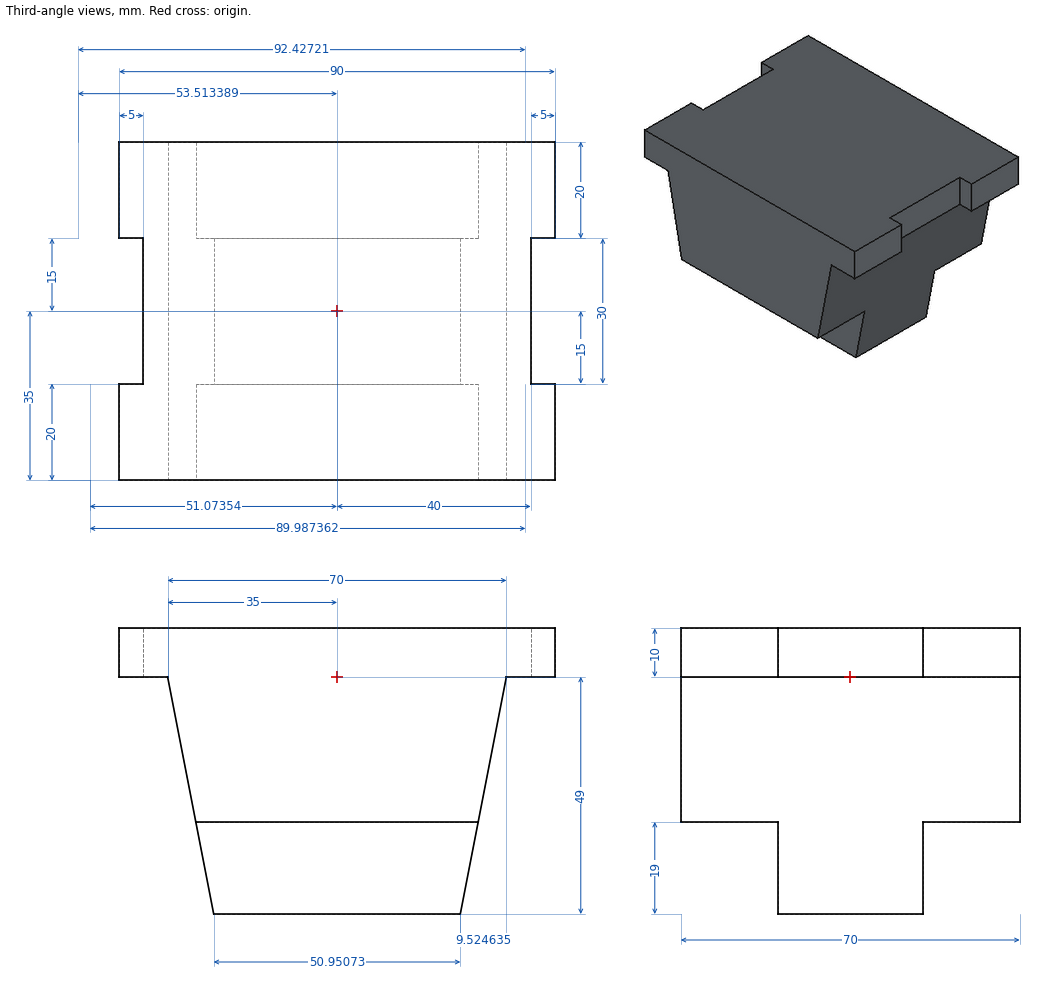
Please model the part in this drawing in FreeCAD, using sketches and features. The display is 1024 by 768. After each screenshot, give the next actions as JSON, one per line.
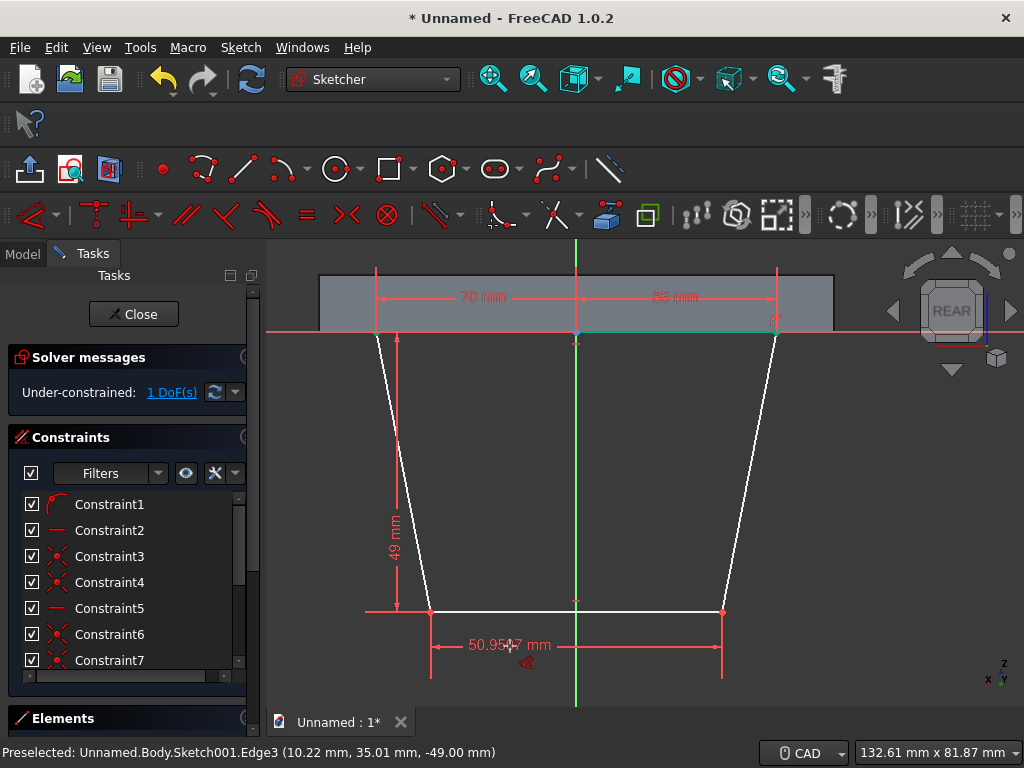
{"action": "left_click", "coordinate": [393, 416]}
{"action": "left_click", "coordinate": [404, 646]}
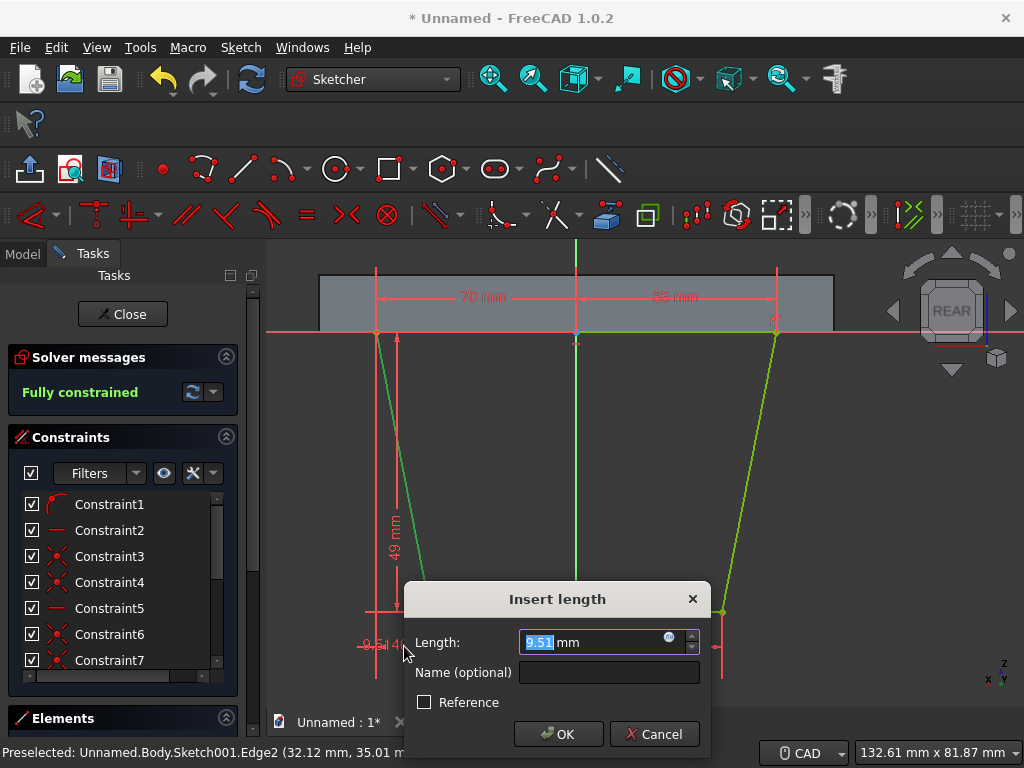
{"action": "type", "text": "9.524635"}
{"action": "key", "text": "Return"}
{"action": "key", "text": "Escape"}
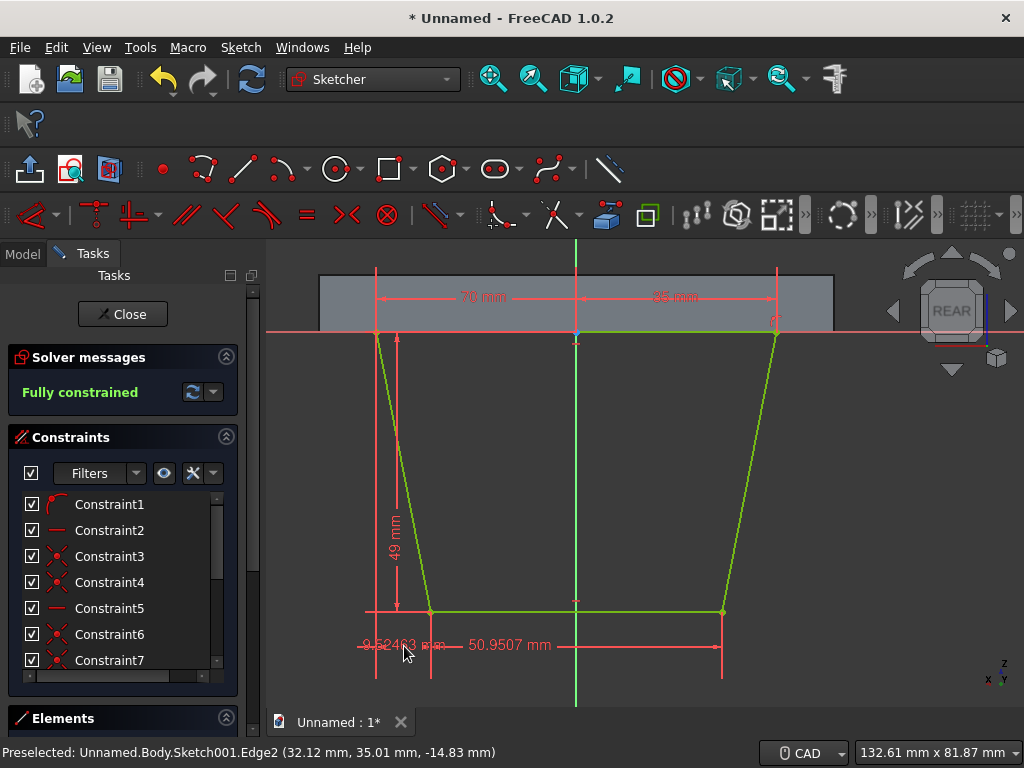
{"action": "left_click", "coordinate": [123, 314]}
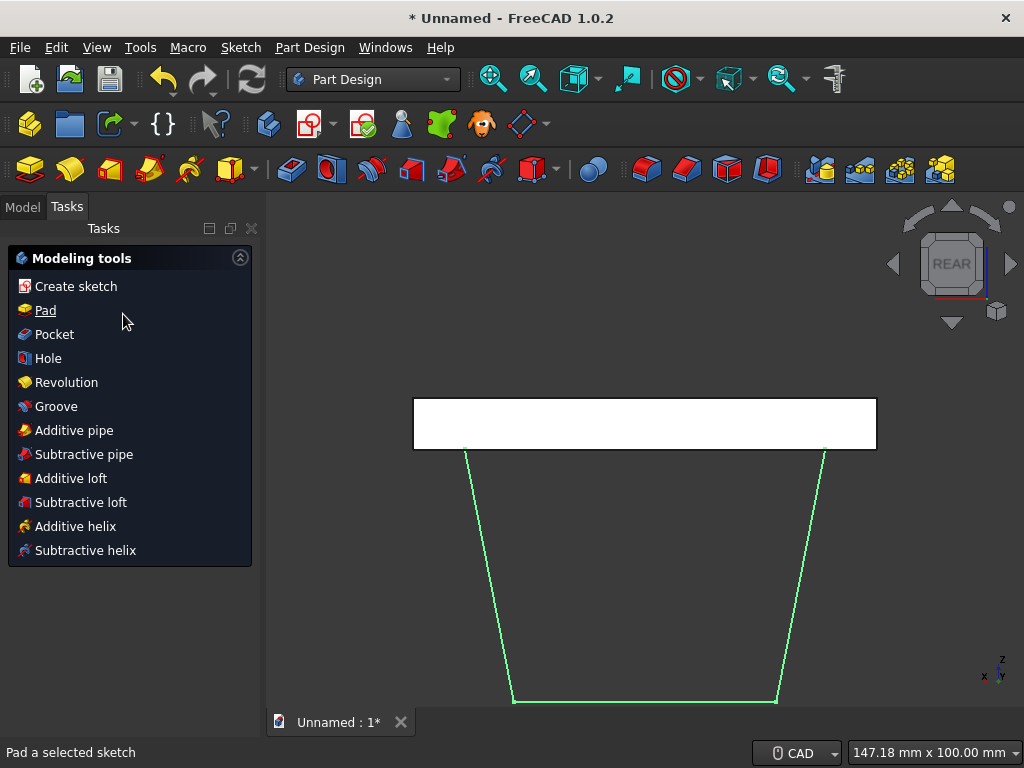
{"action": "left_click", "coordinate": [30, 170]}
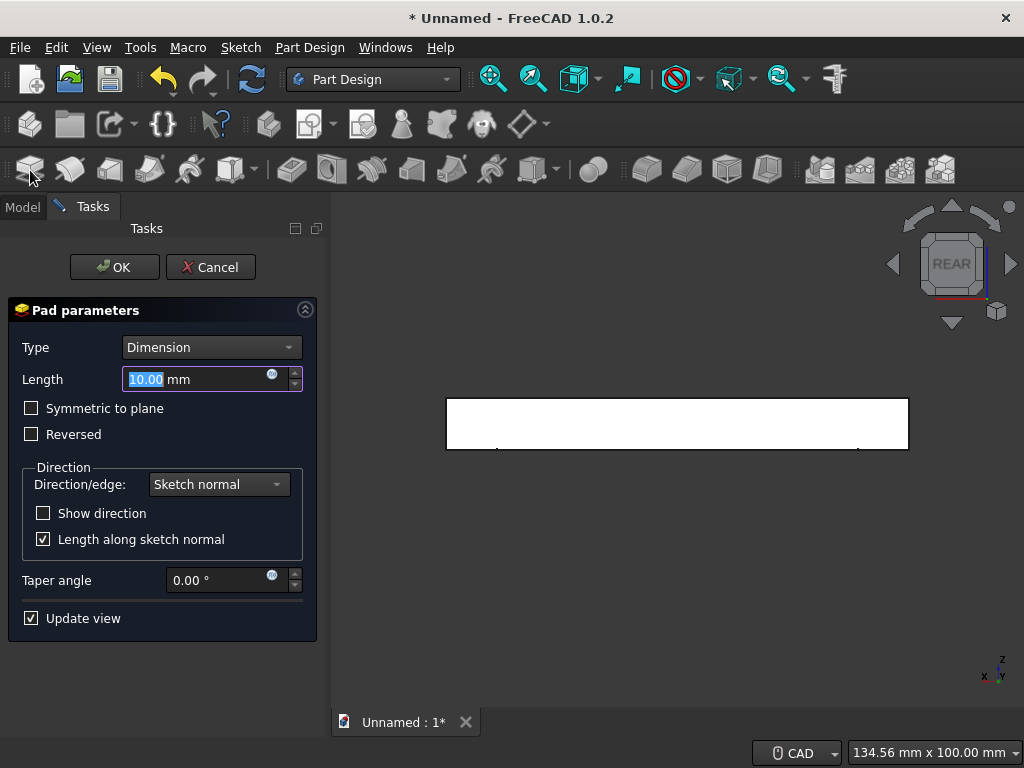
{"action": "type", "text": "70"}
{"action": "key", "text": "Tab"}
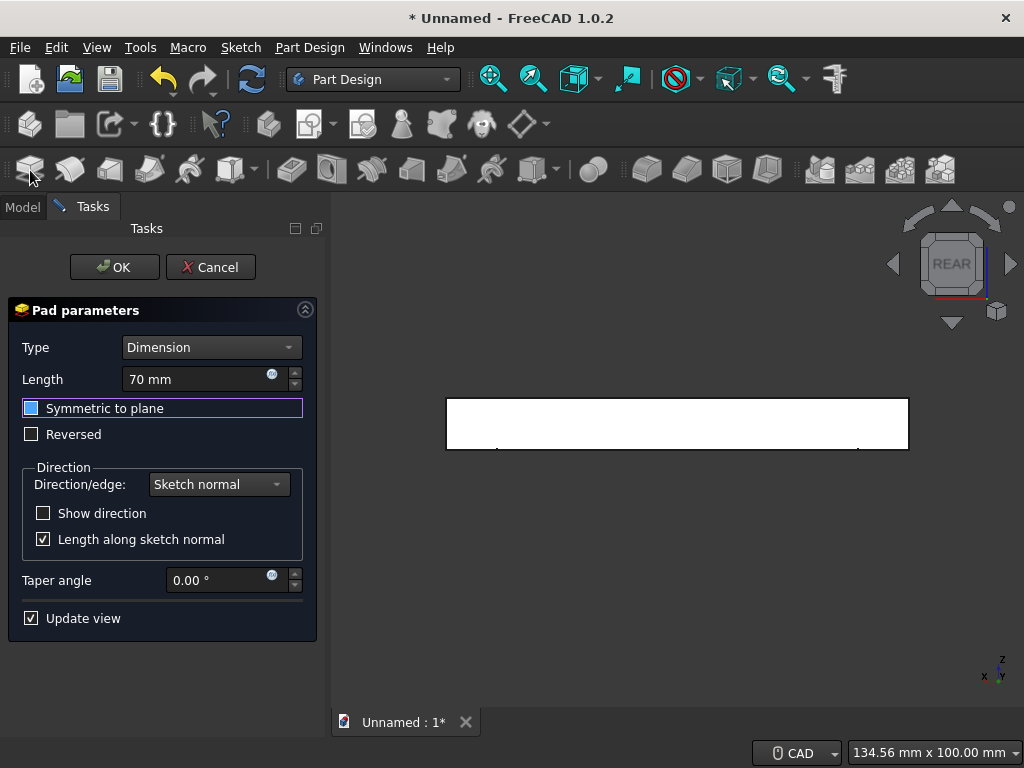
{"action": "left_click", "coordinate": [30, 434]}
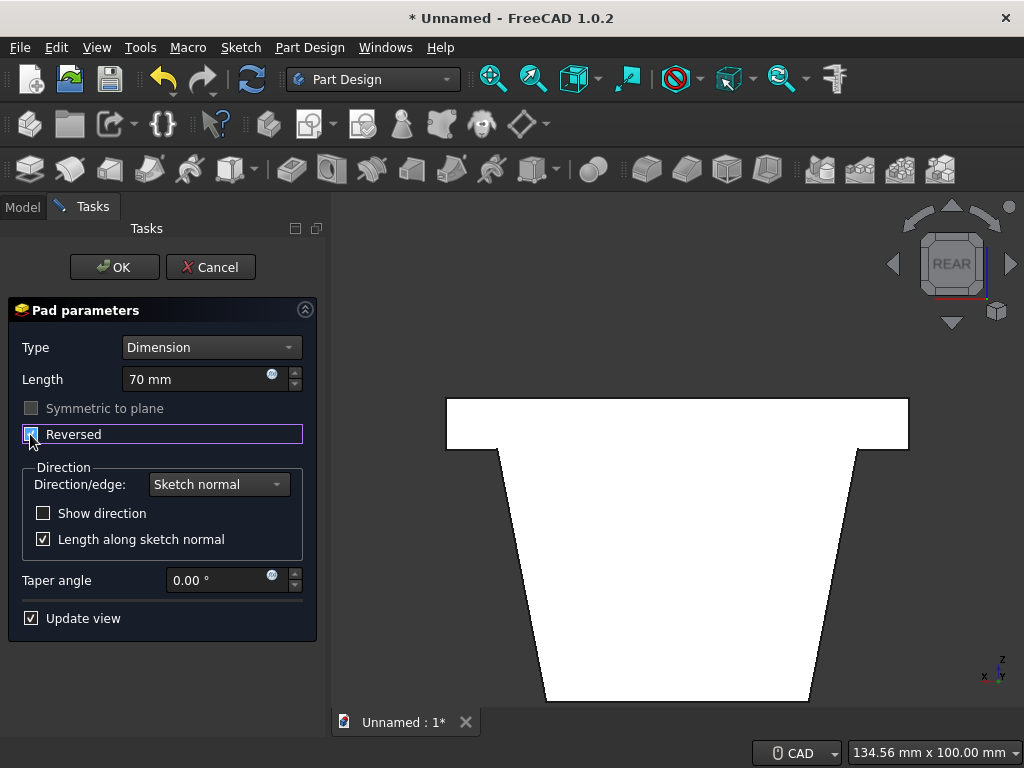
{"action": "left_click", "coordinate": [115, 267]}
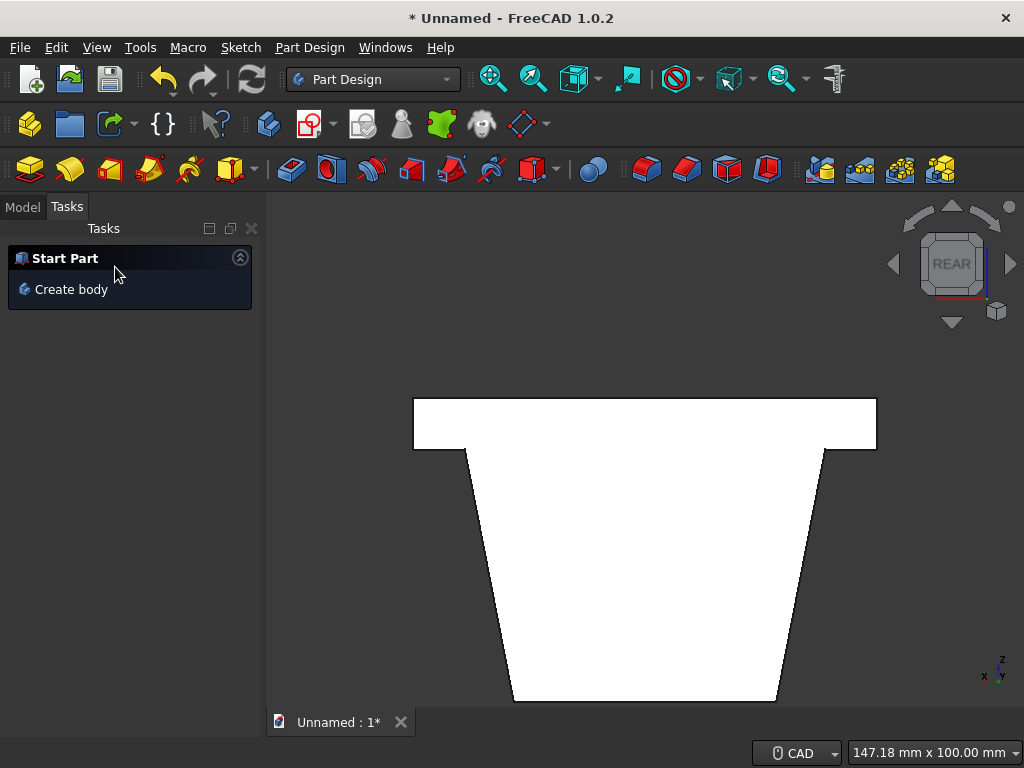
{"action": "key", "text": "5"}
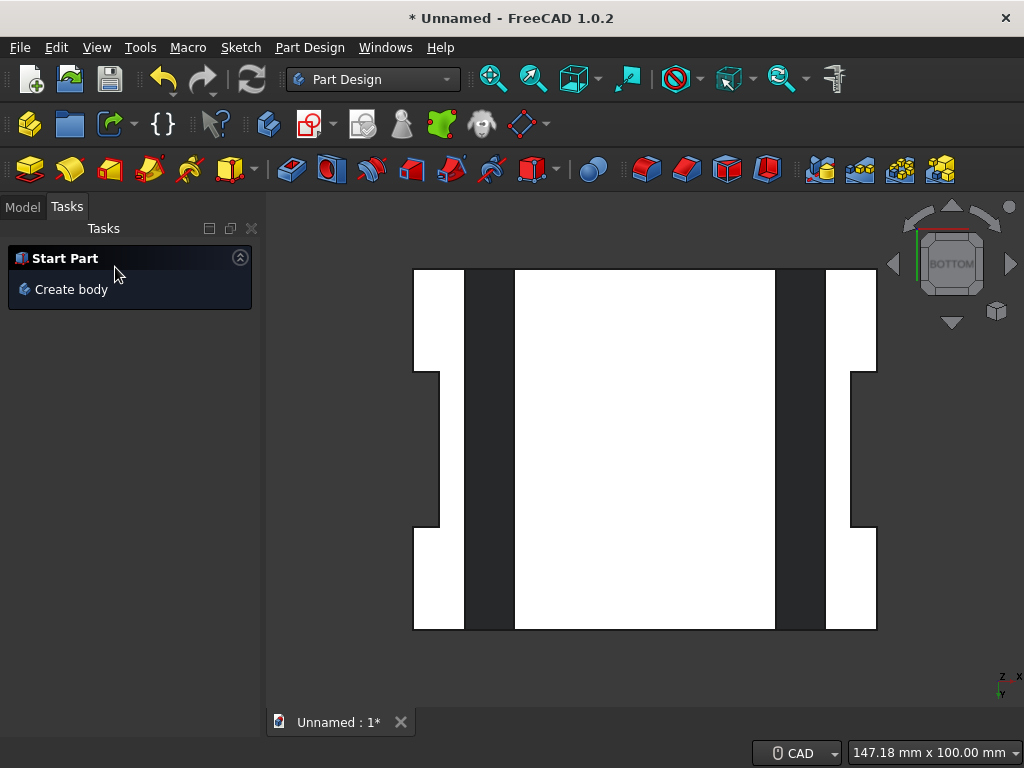
{"action": "left_click", "coordinate": [645, 449]}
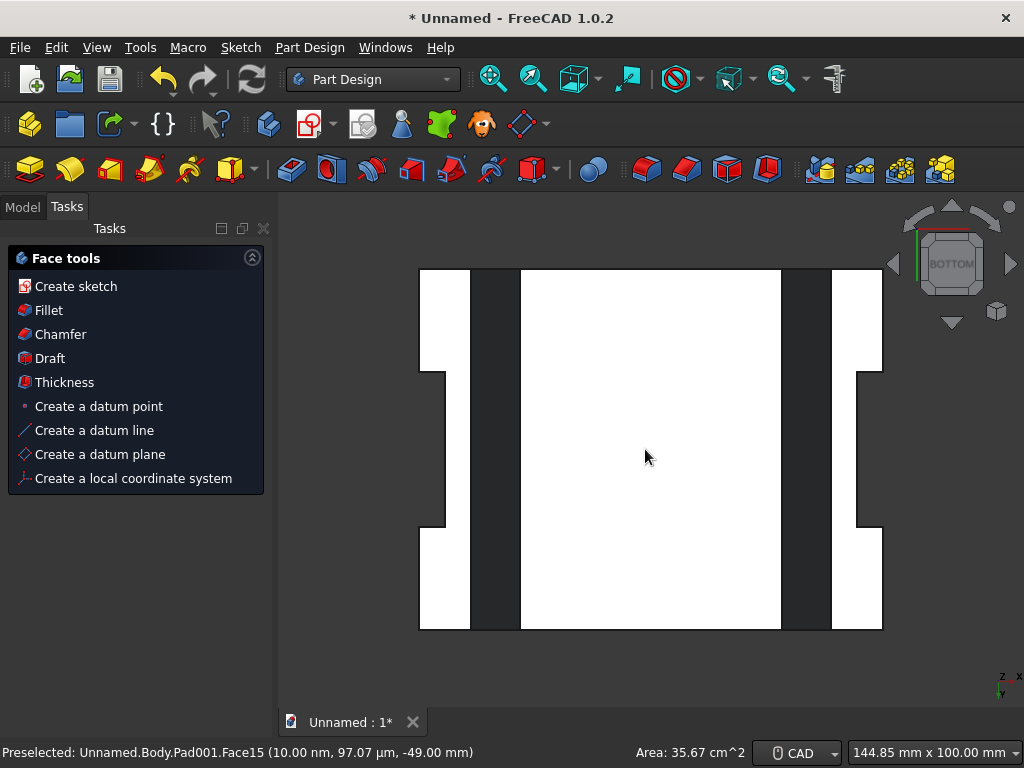
{"action": "left_click", "coordinate": [310, 124]}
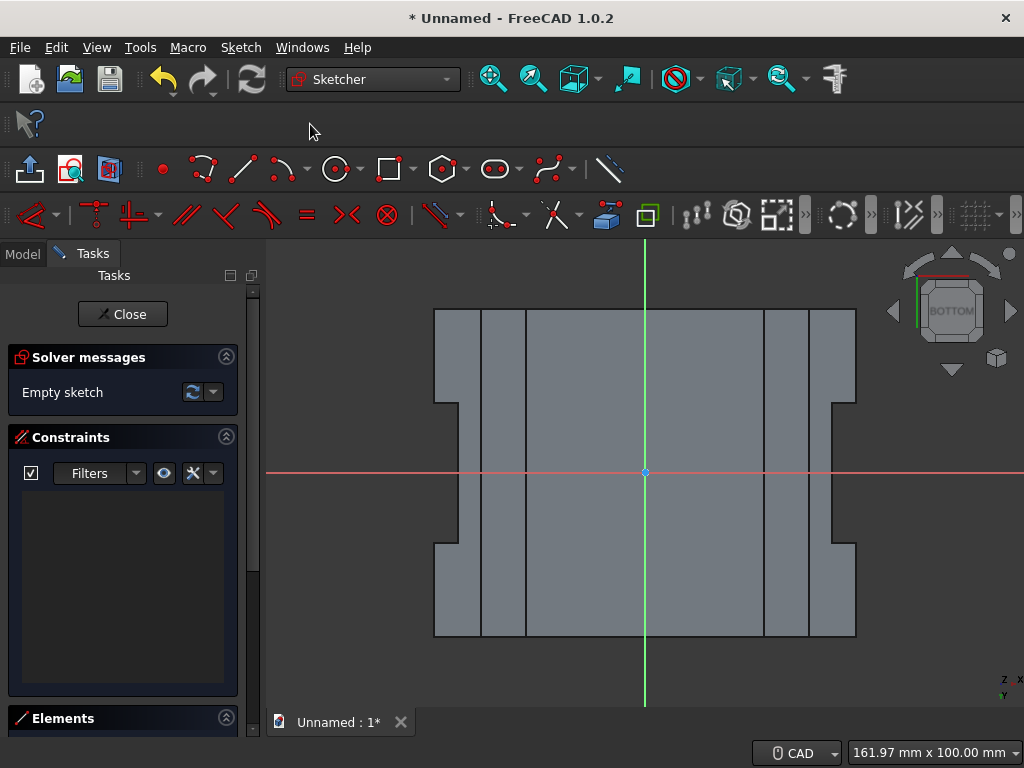
{"action": "left_click", "coordinate": [390, 170]}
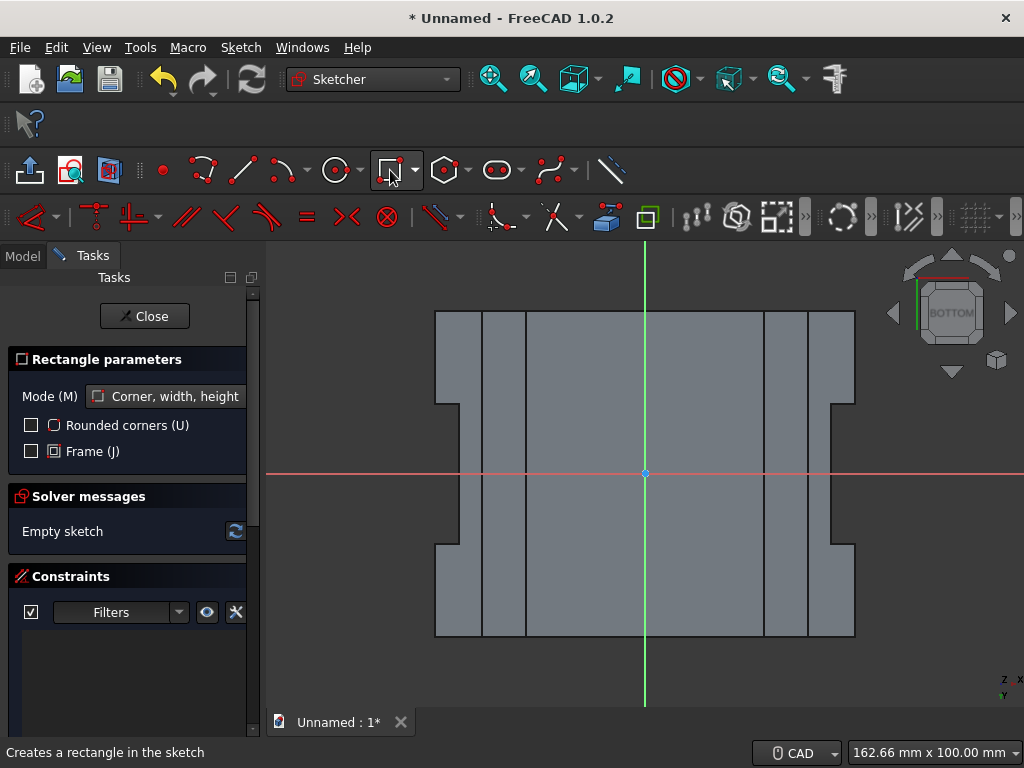
{"action": "left_click", "coordinate": [396, 544]}
{"action": "mouse_move", "coordinate": [826, 637]}